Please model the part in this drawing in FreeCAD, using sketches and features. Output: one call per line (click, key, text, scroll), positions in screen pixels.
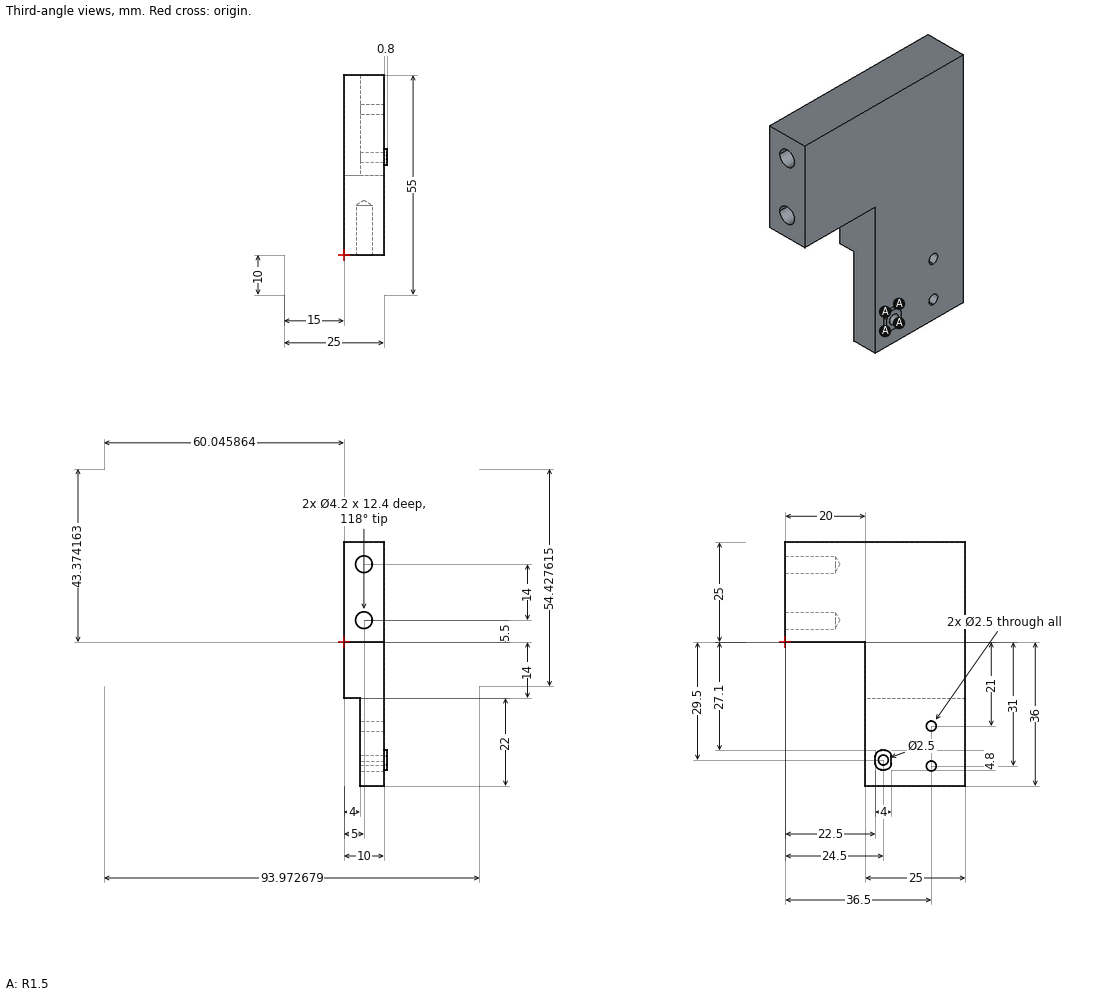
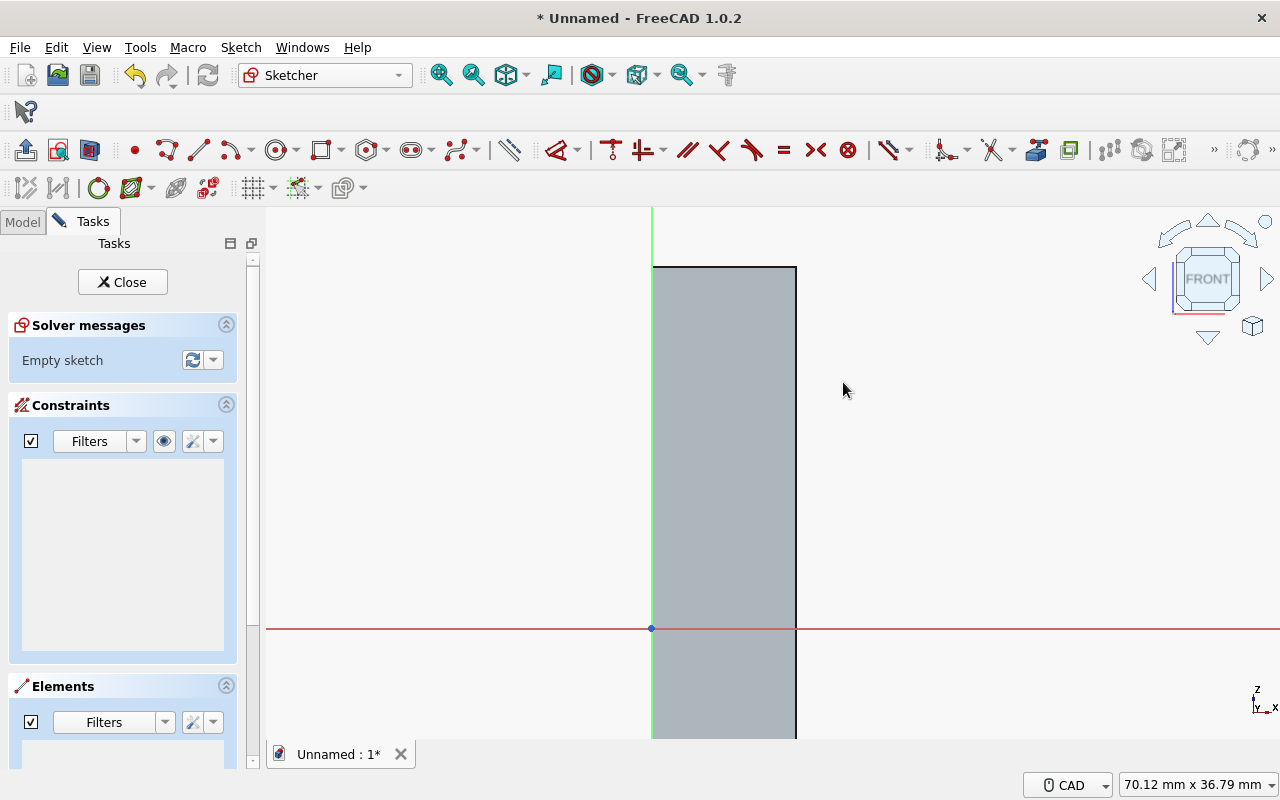
click(276, 150)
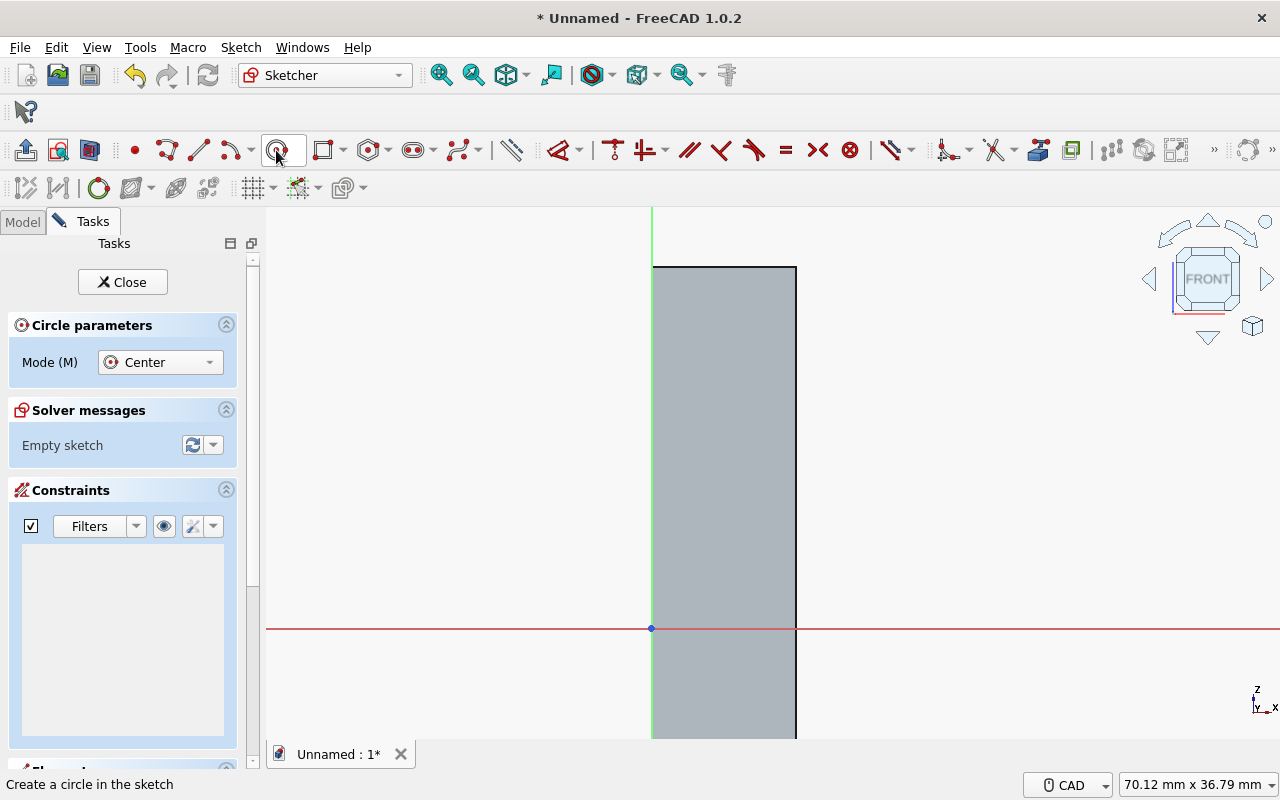
click(724, 549)
move(746, 528)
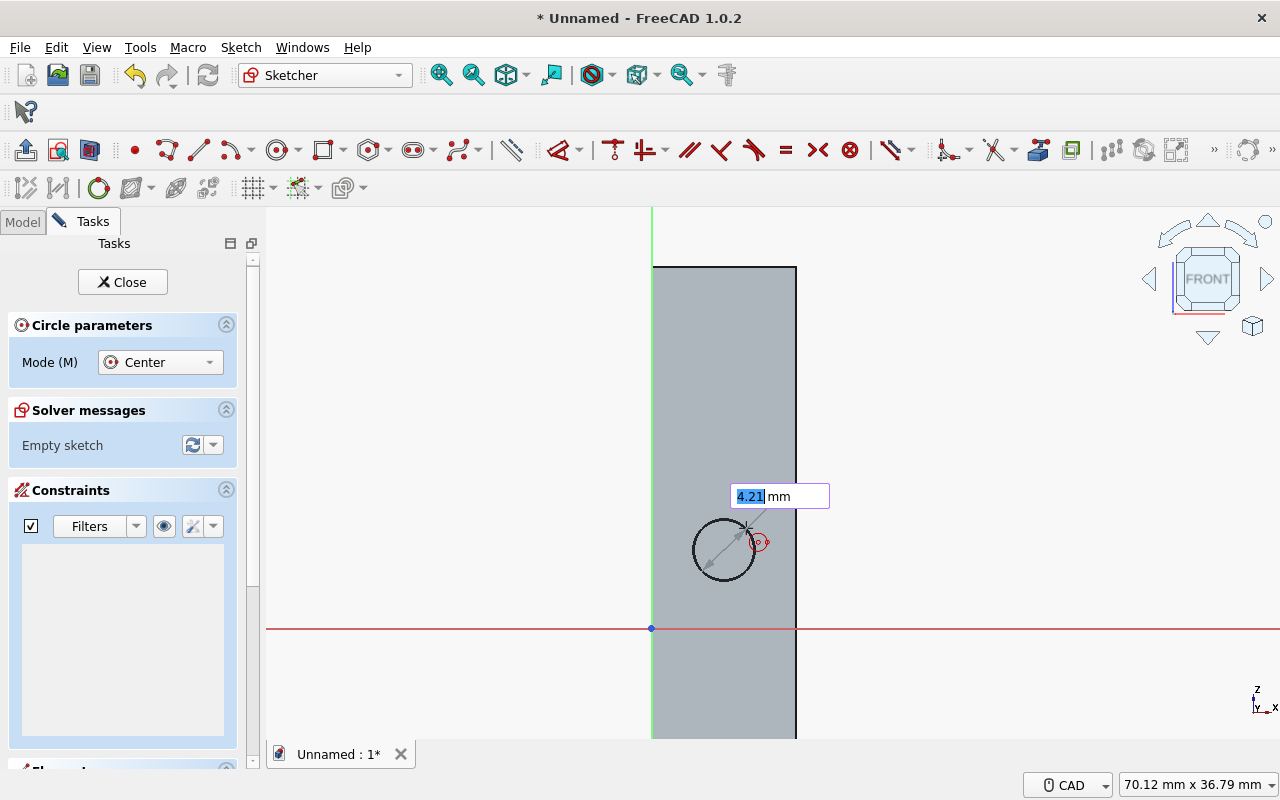
text(4.2)
key(Return)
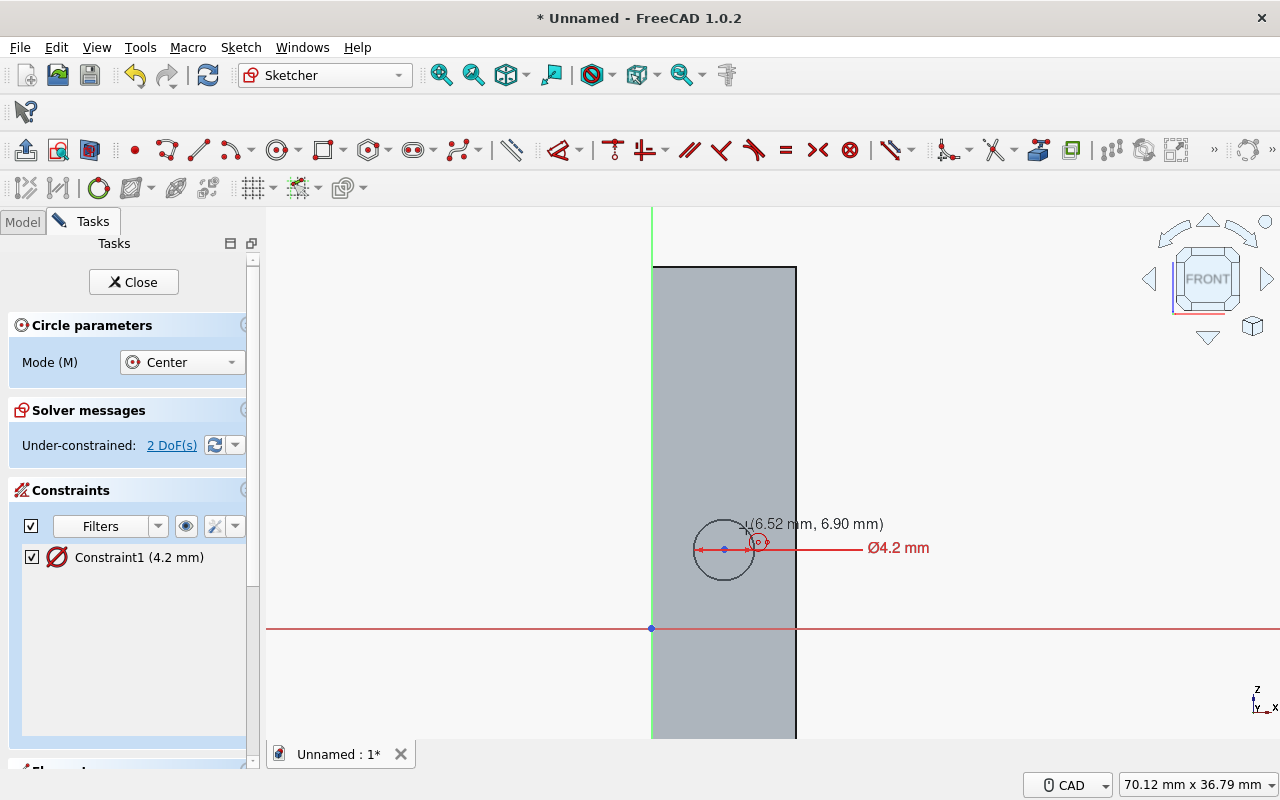
click(724, 347)
move(746, 325)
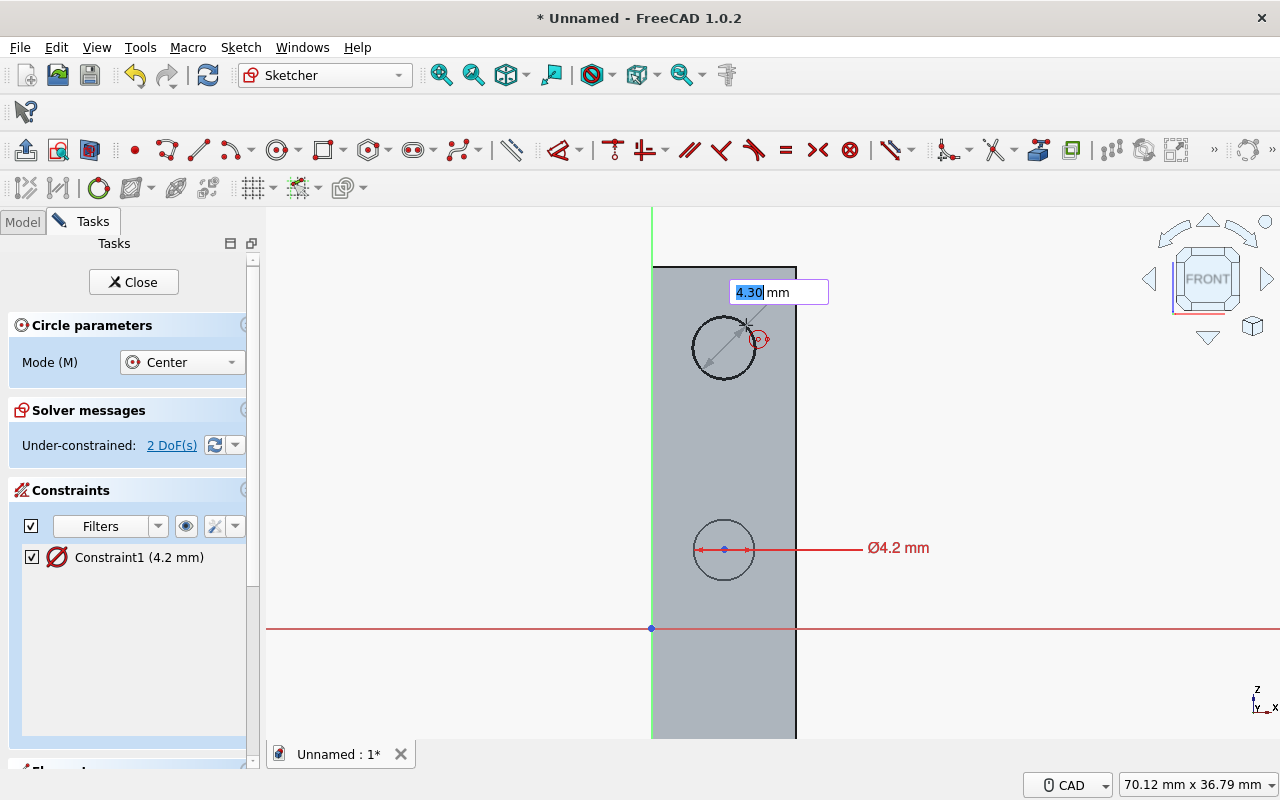
text(4.2)
key(Return)
key(Escape)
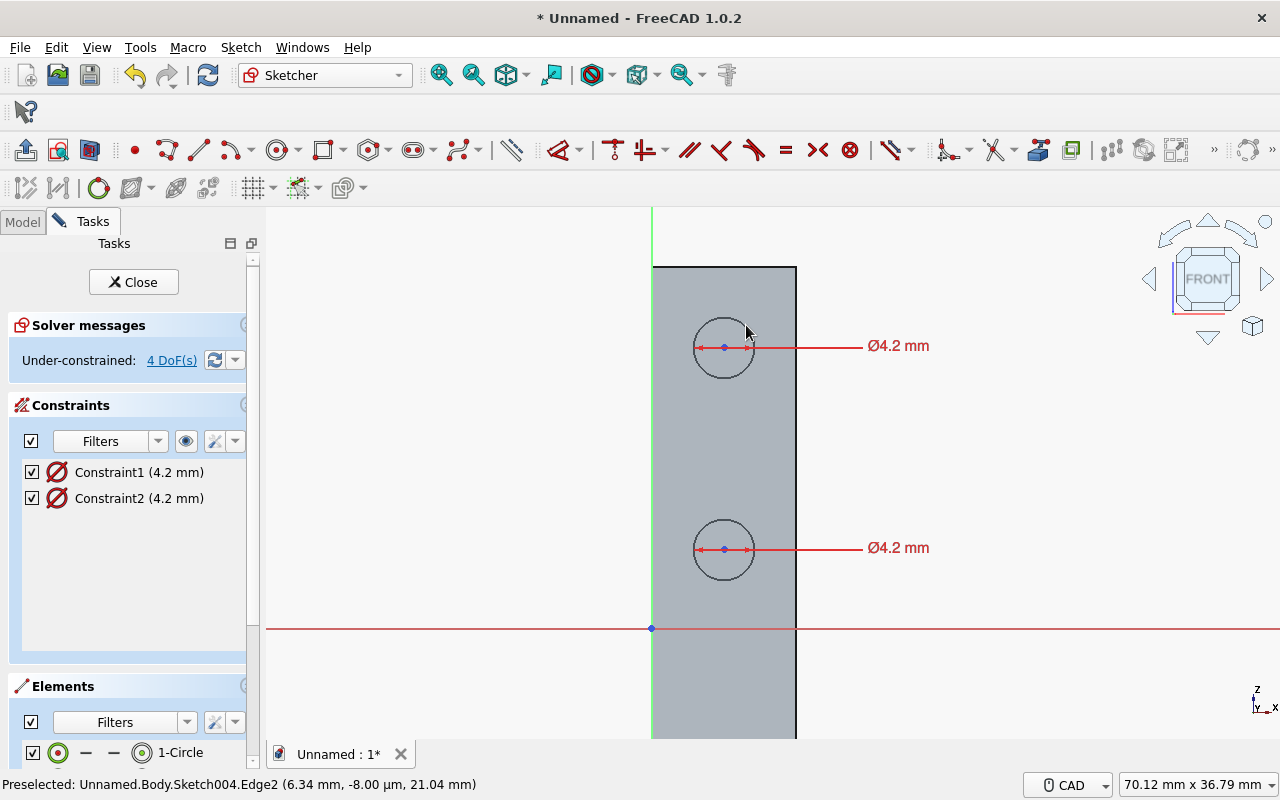
click(724, 550)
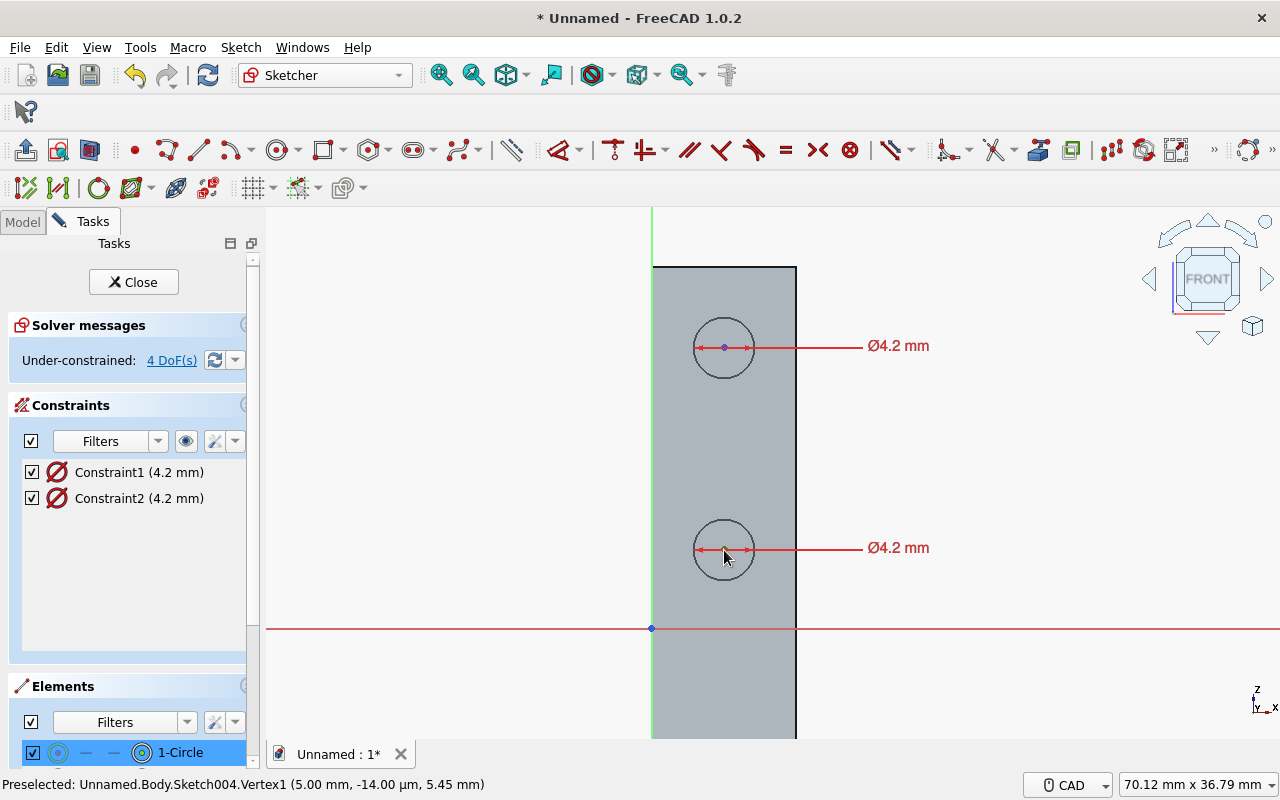
click(724, 348)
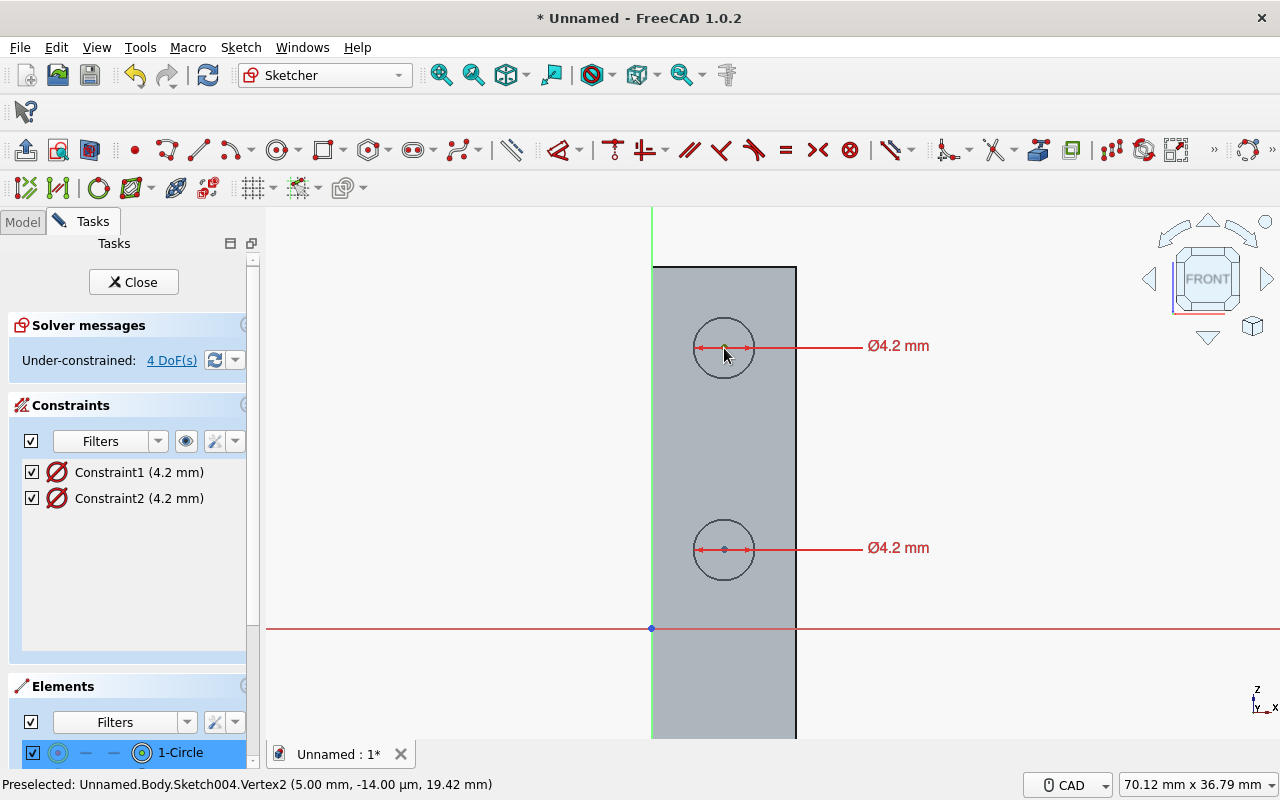
click(668, 150)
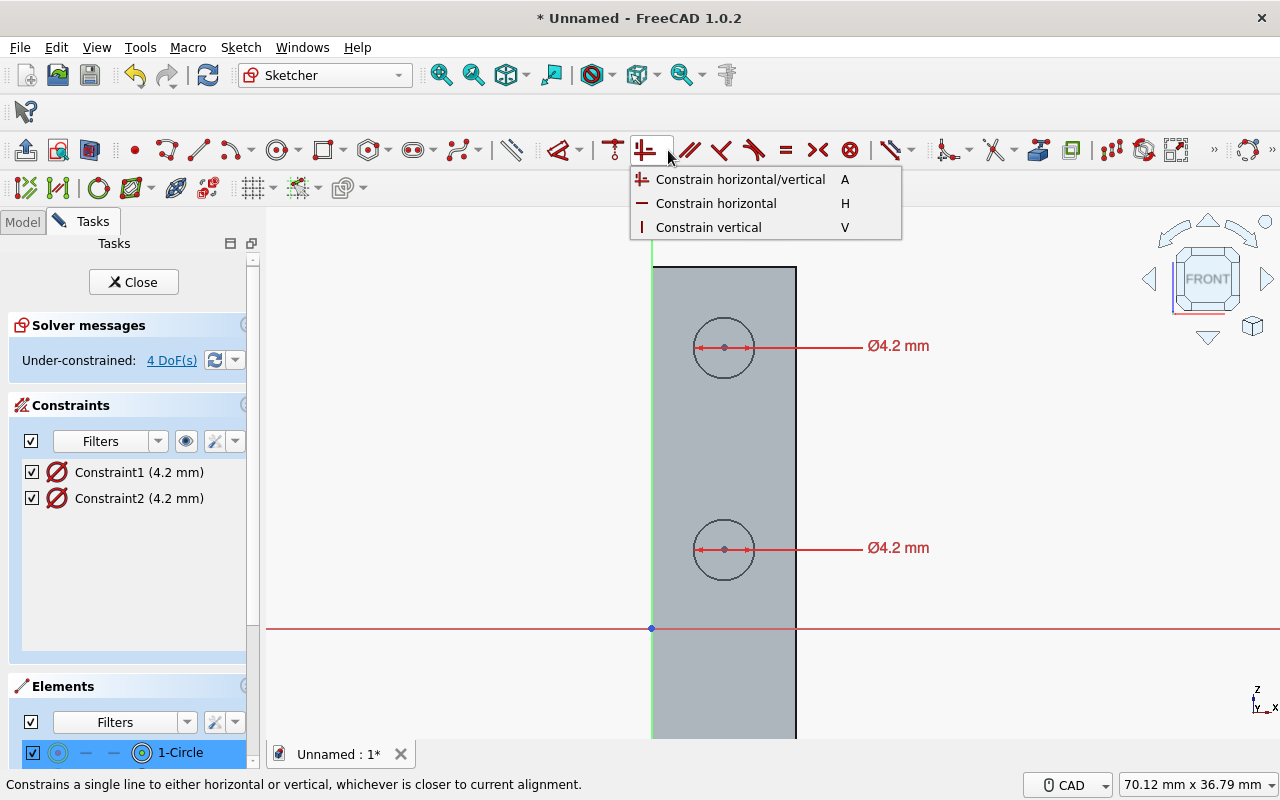
click(766, 227)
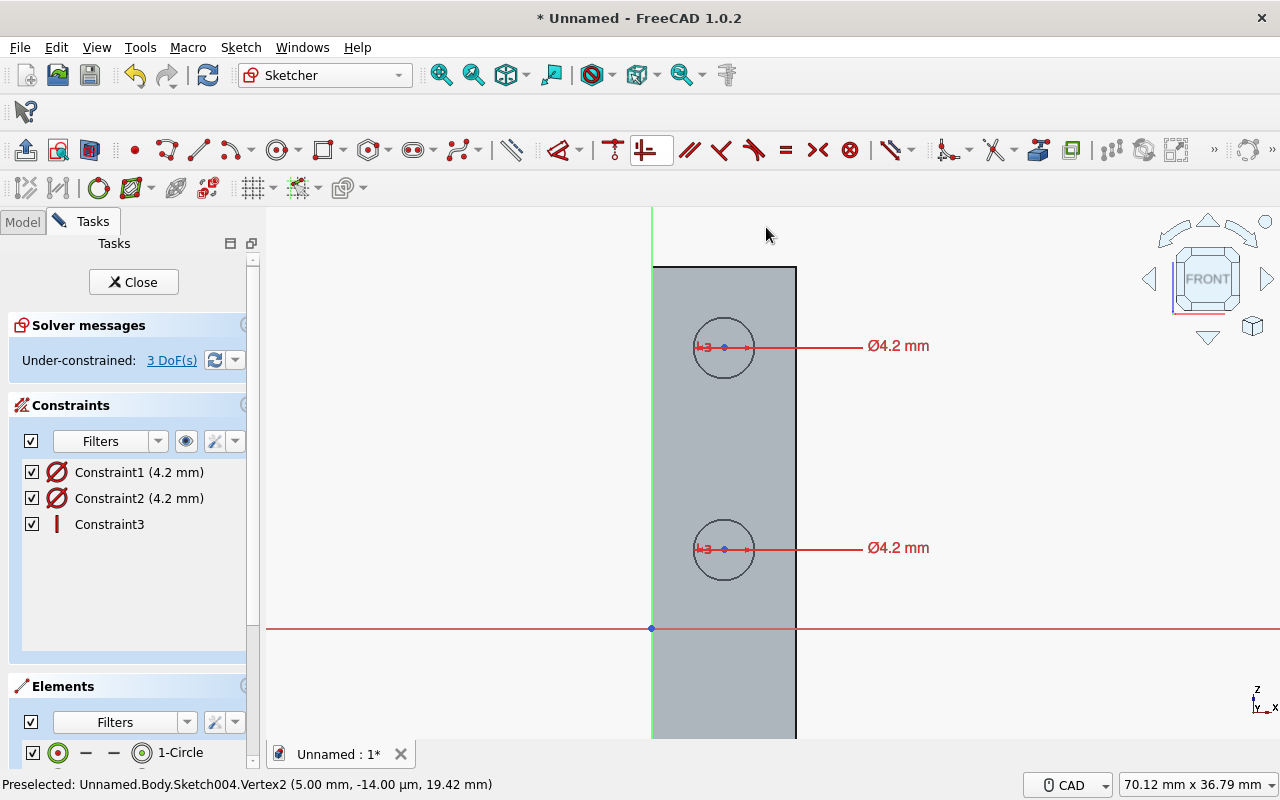
click(558, 150)